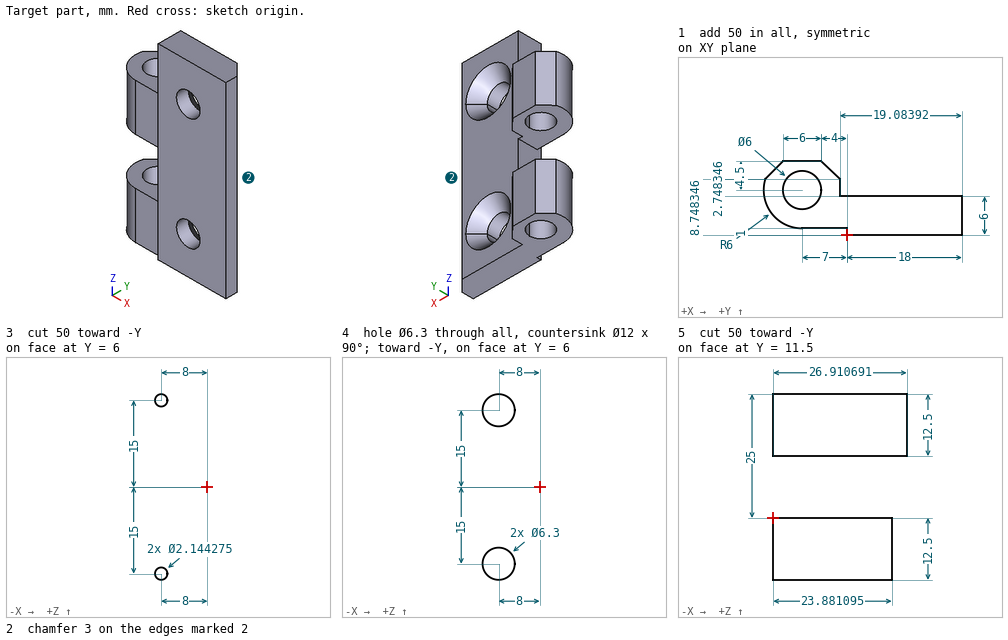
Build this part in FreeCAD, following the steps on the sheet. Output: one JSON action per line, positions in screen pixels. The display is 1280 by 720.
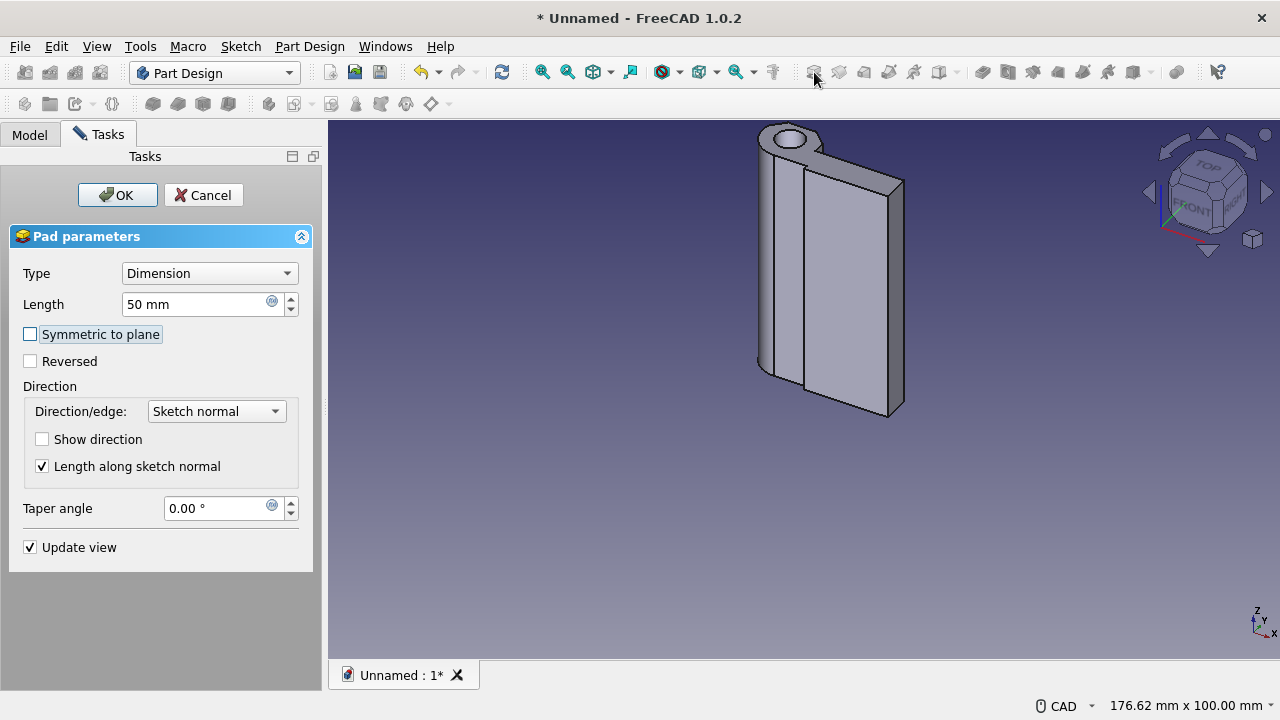
{"action": "left_click", "coordinate": [31, 334]}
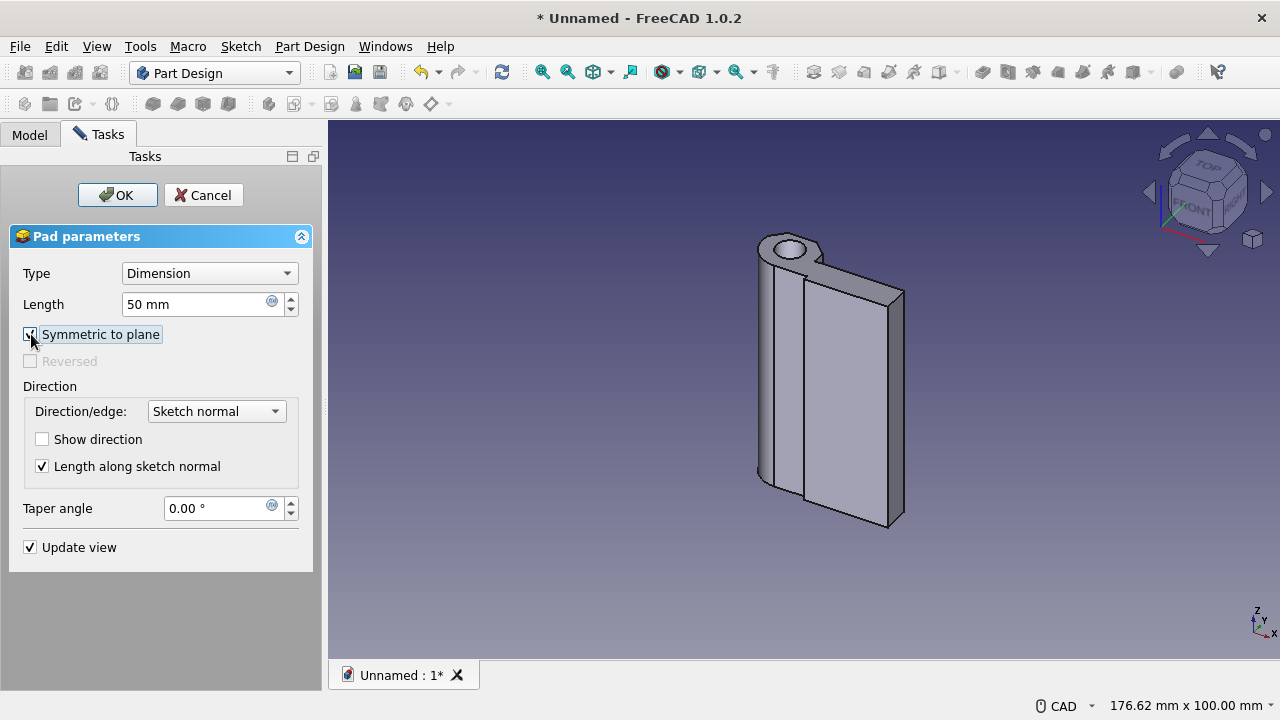
{"action": "left_click", "coordinate": [118, 195]}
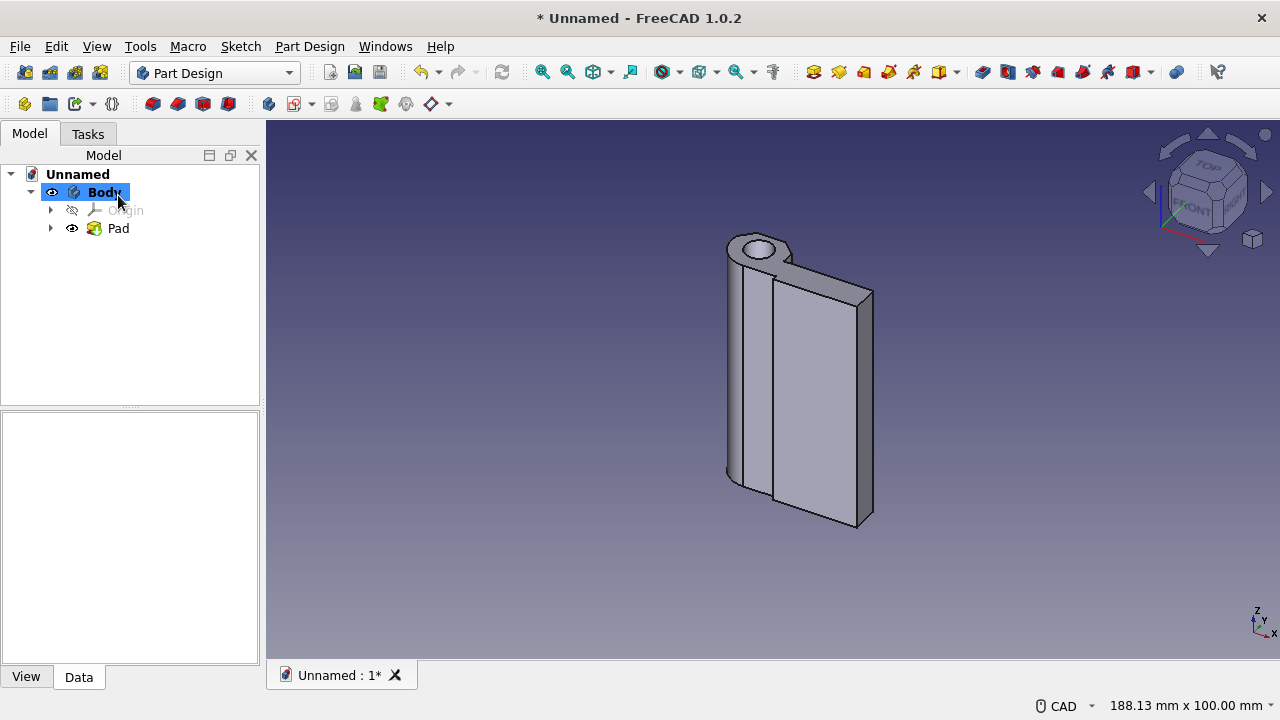
{"action": "key", "text": "0"}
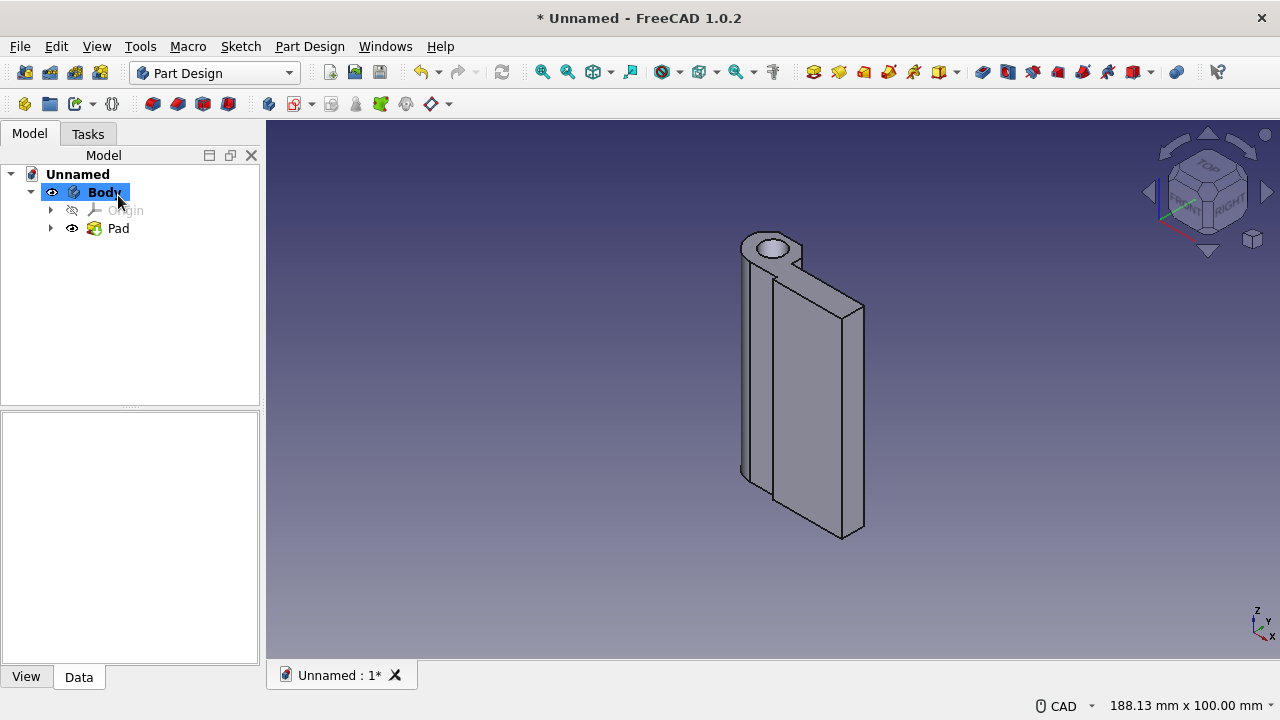
{"action": "key", "text": "2"}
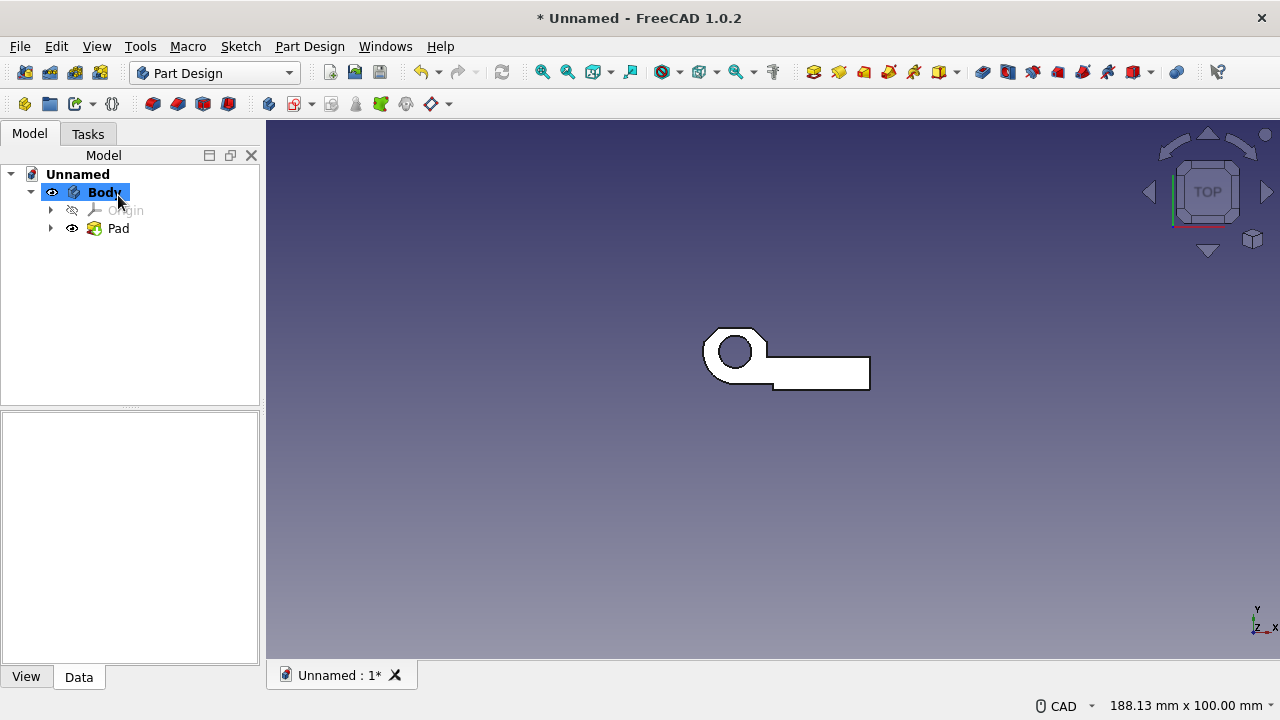
{"action": "left_click", "coordinate": [543, 72]}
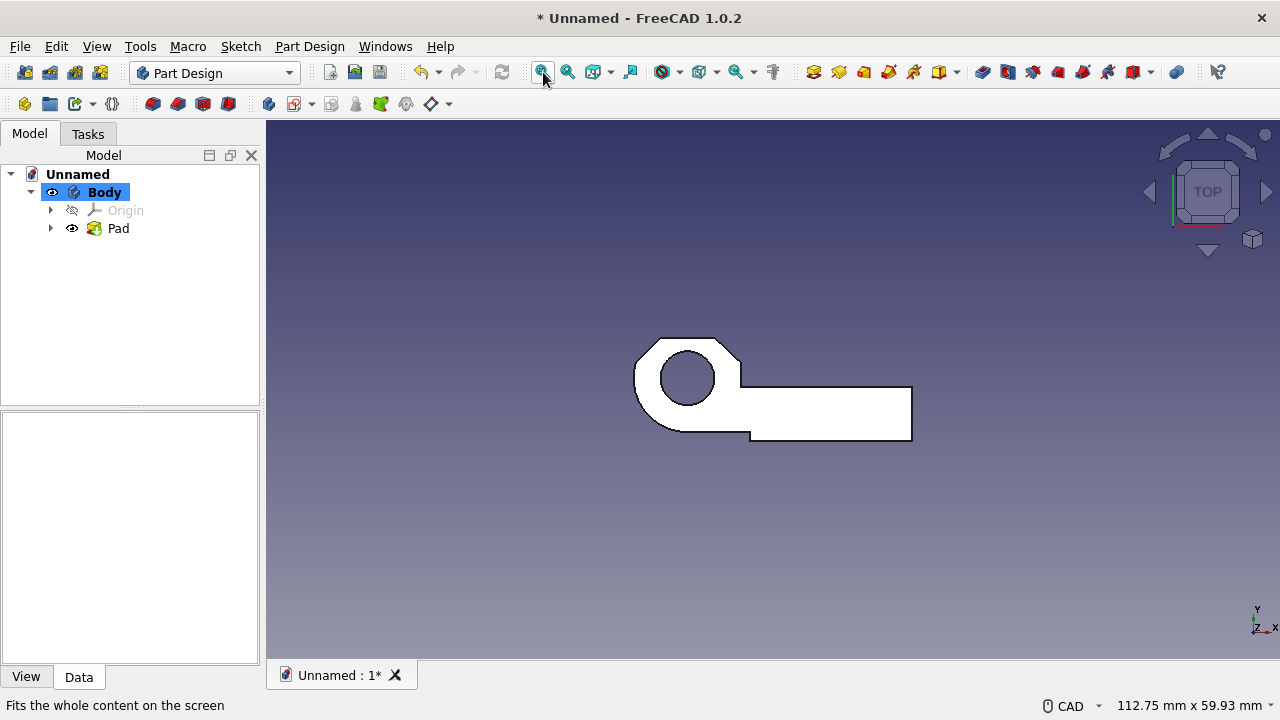
{"action": "key", "text": "1"}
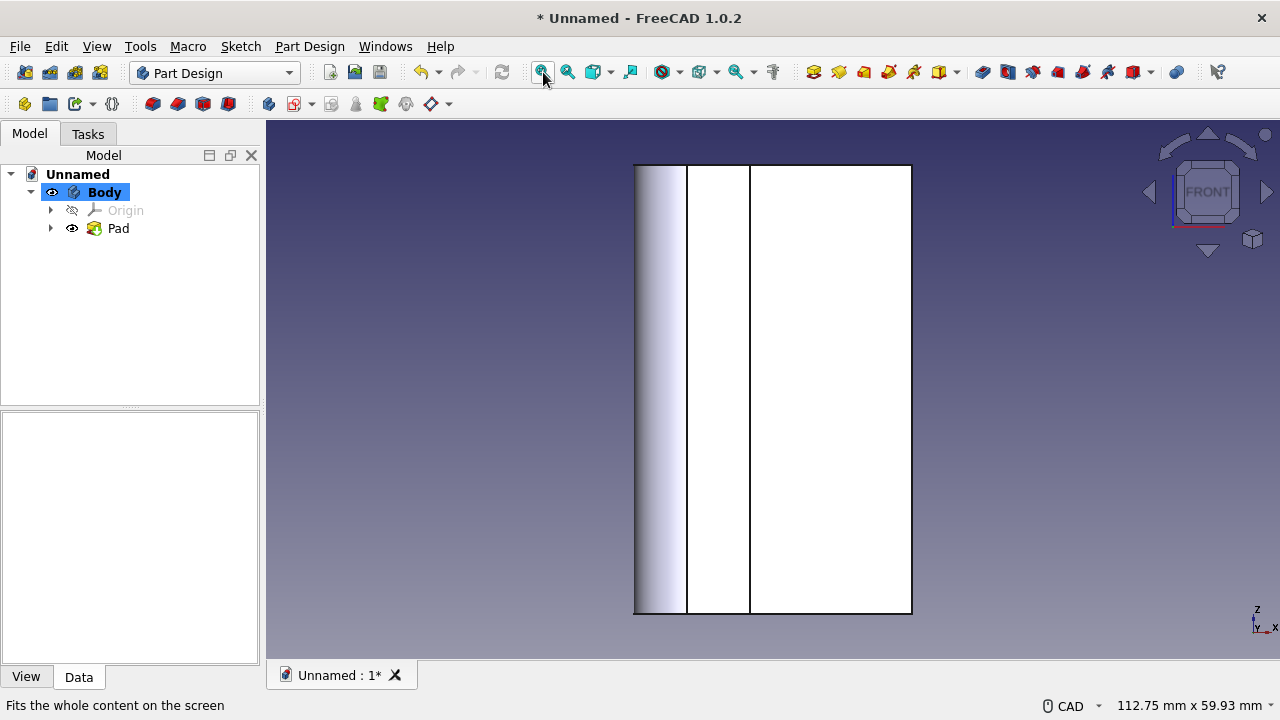
{"action": "key", "text": "3"}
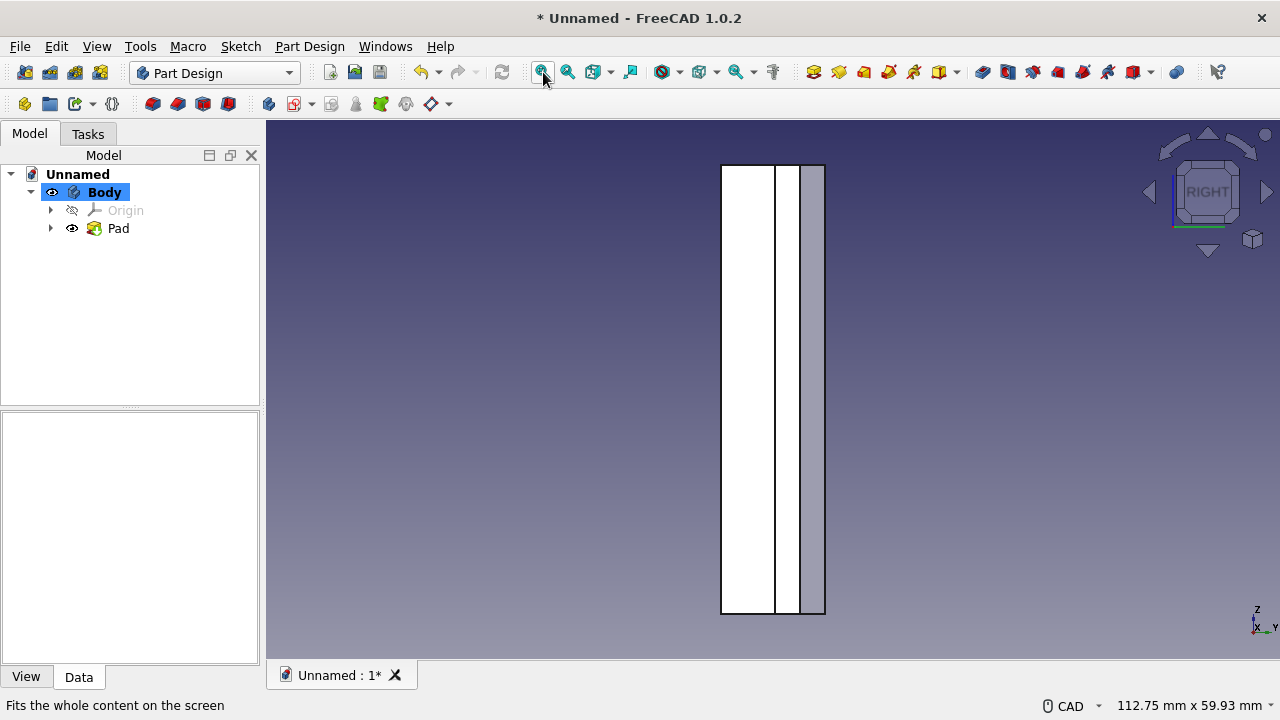
{"action": "left_click", "coordinate": [775, 388]}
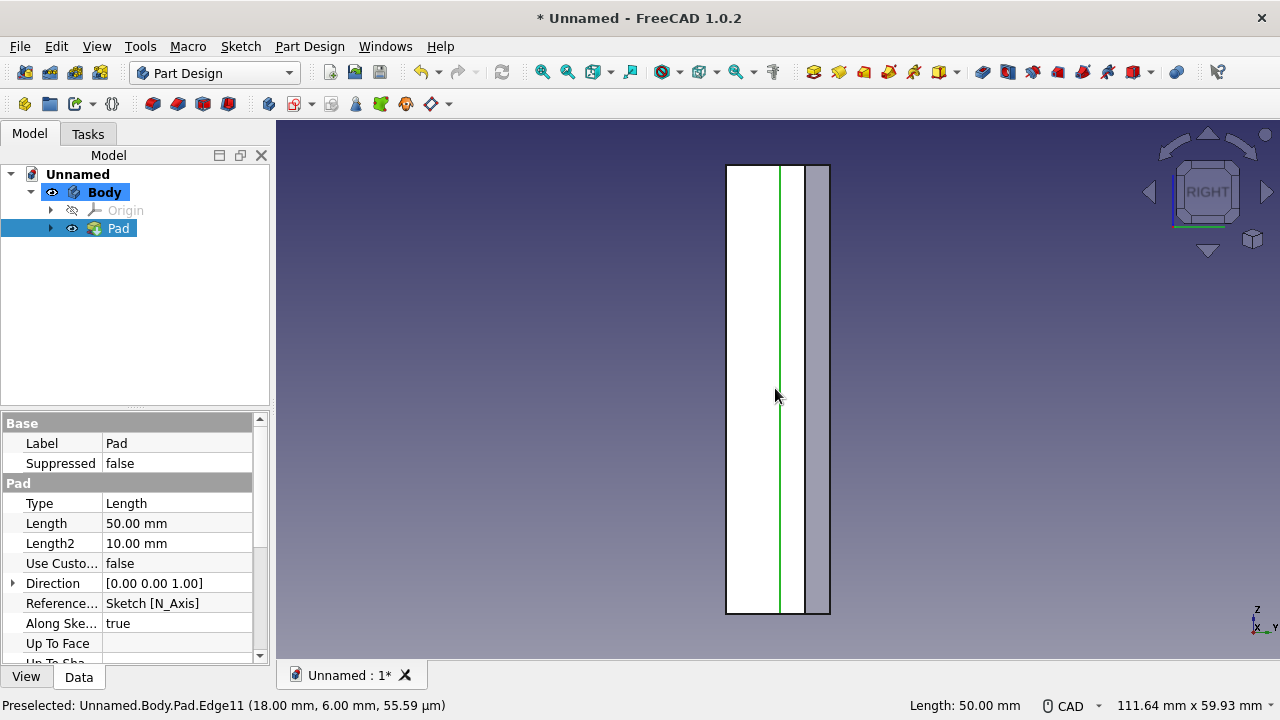
{"action": "left_click", "coordinate": [178, 104]}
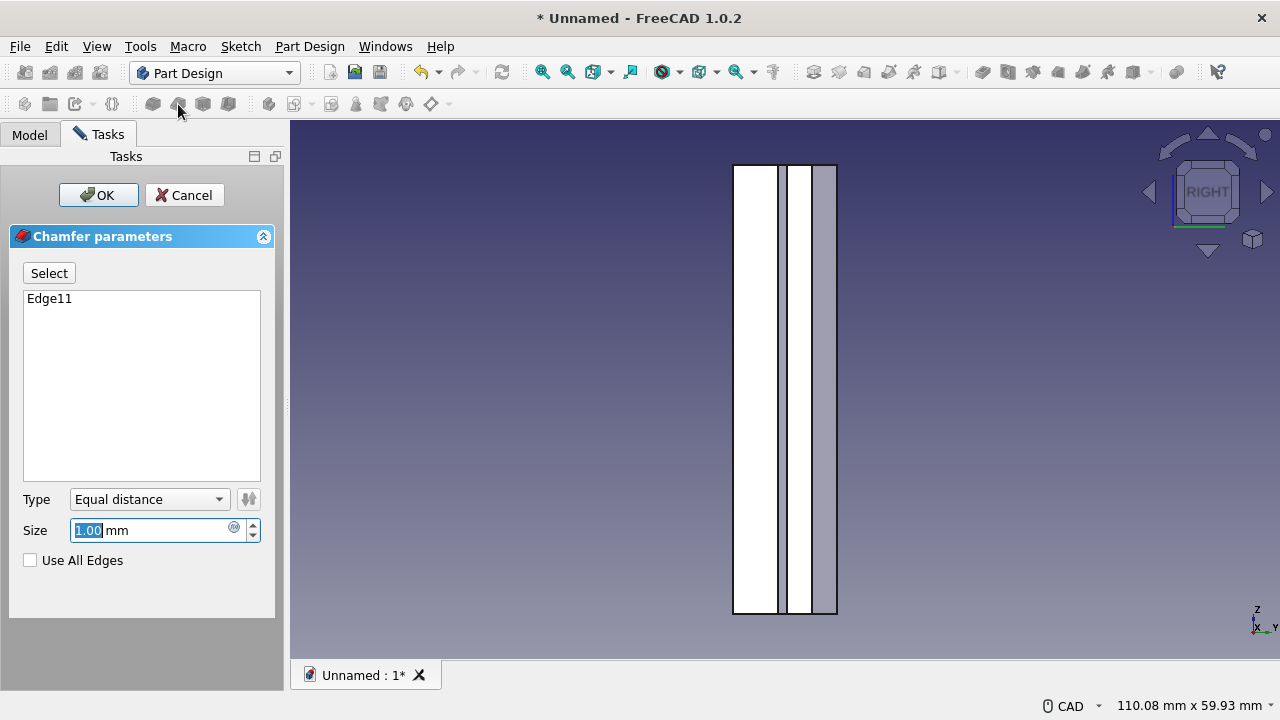
{"action": "type", "text": "3"}
{"action": "key", "text": "Tab"}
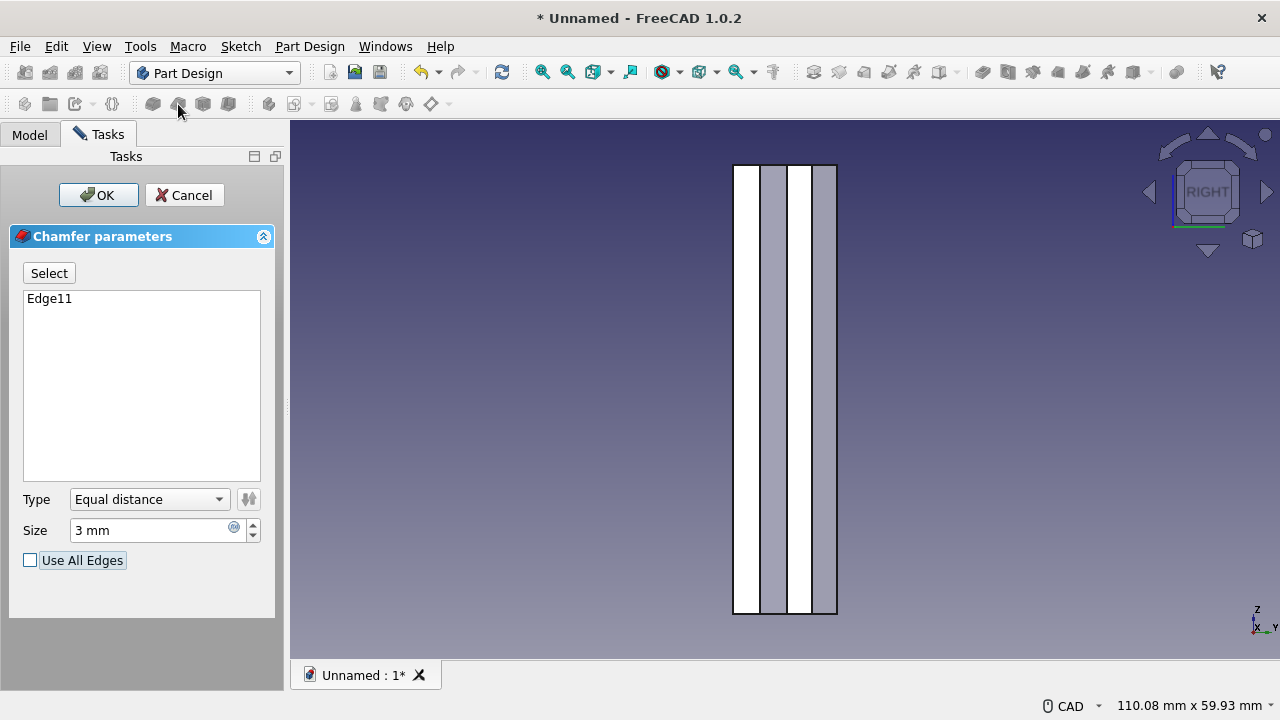
{"action": "left_click", "coordinate": [99, 195]}